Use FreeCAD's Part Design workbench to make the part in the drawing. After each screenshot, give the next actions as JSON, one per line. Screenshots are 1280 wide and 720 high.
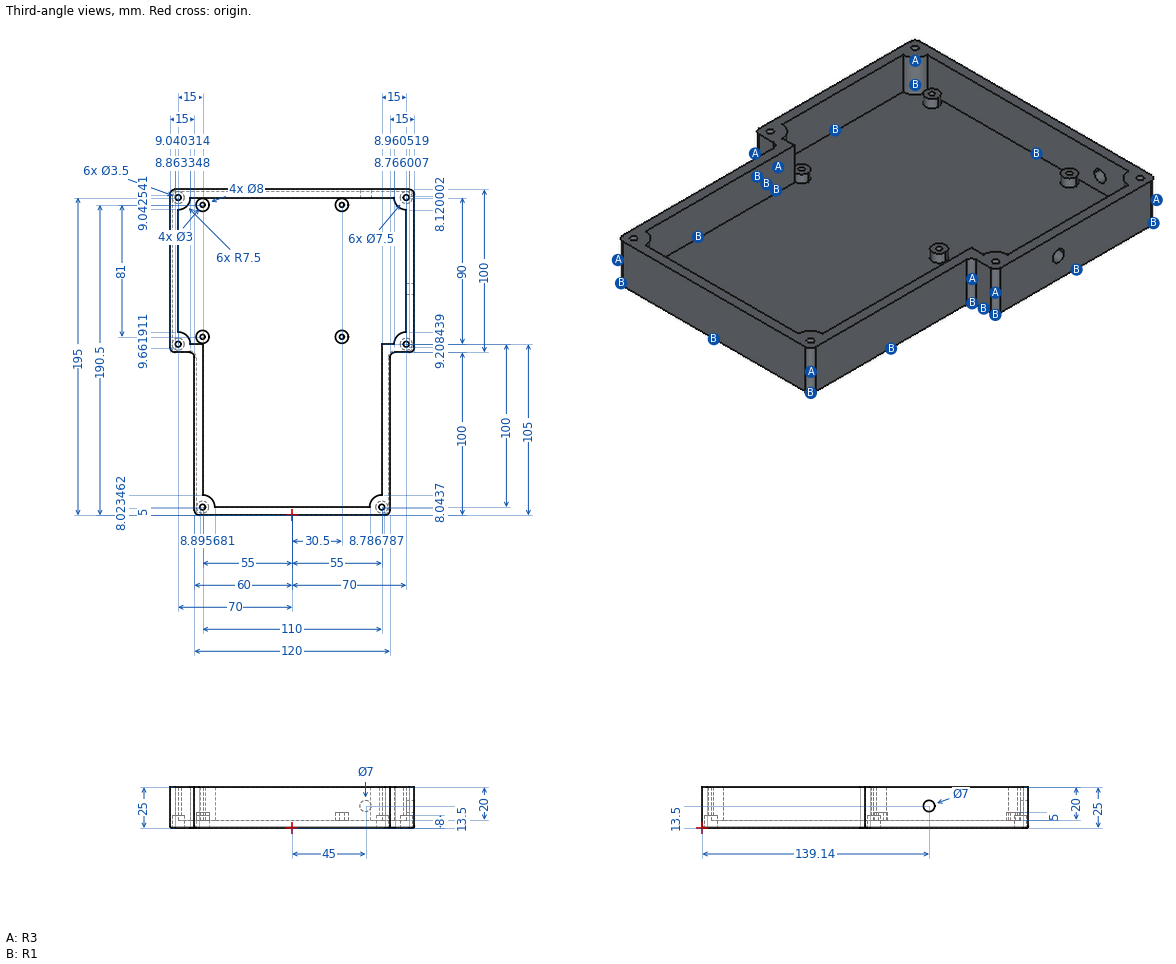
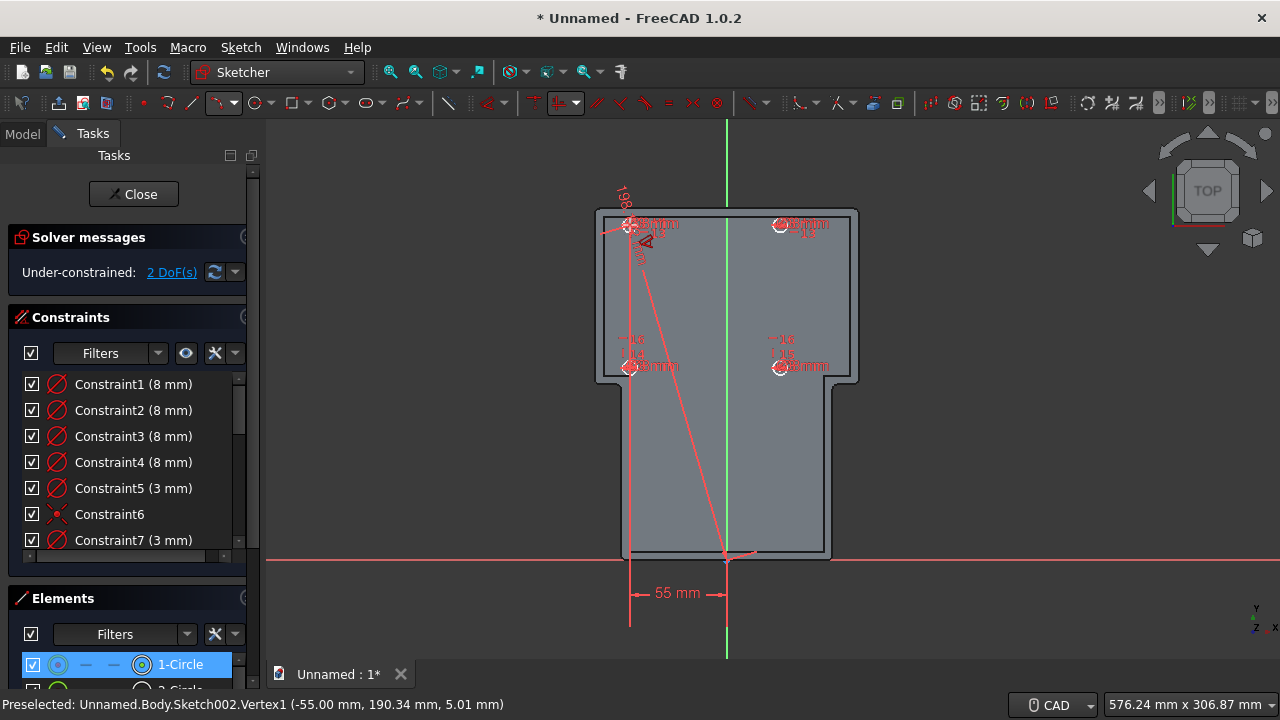
{"action": "left_click", "coordinate": [630, 368]}
{"action": "left_click", "coordinate": [596, 297]}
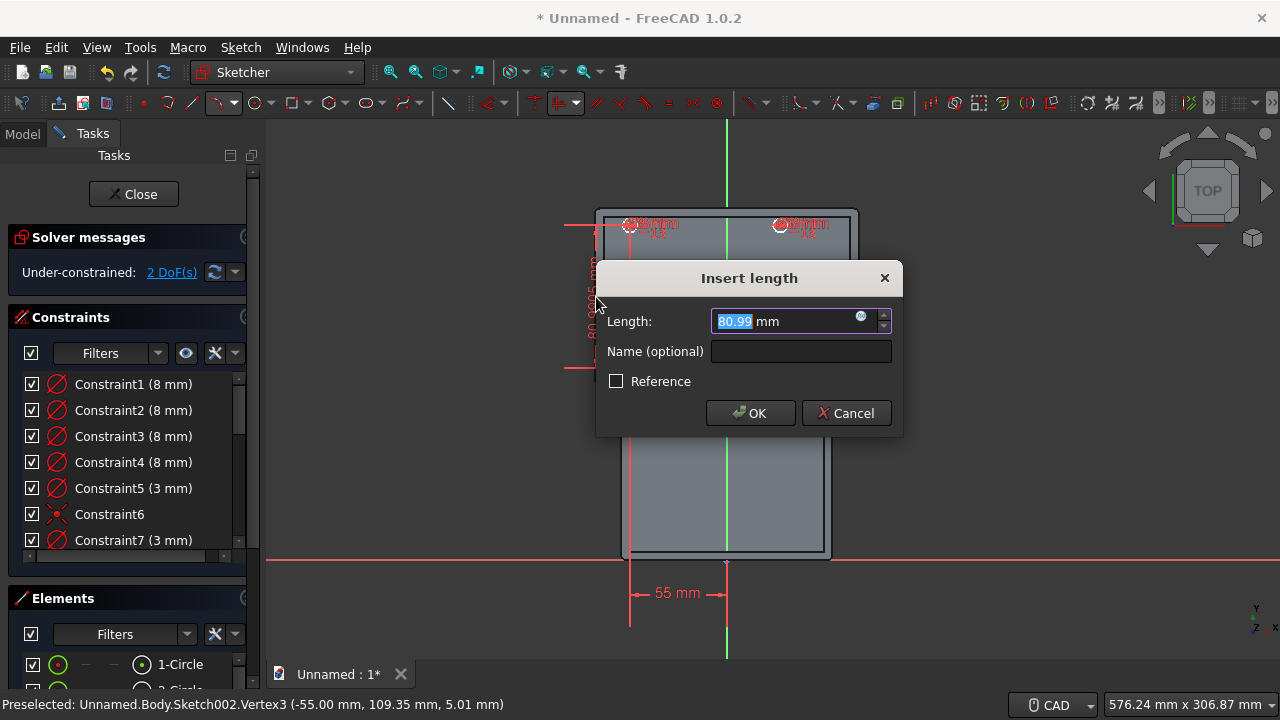
{"action": "type", "text": "81"}
{"action": "key", "text": "Return"}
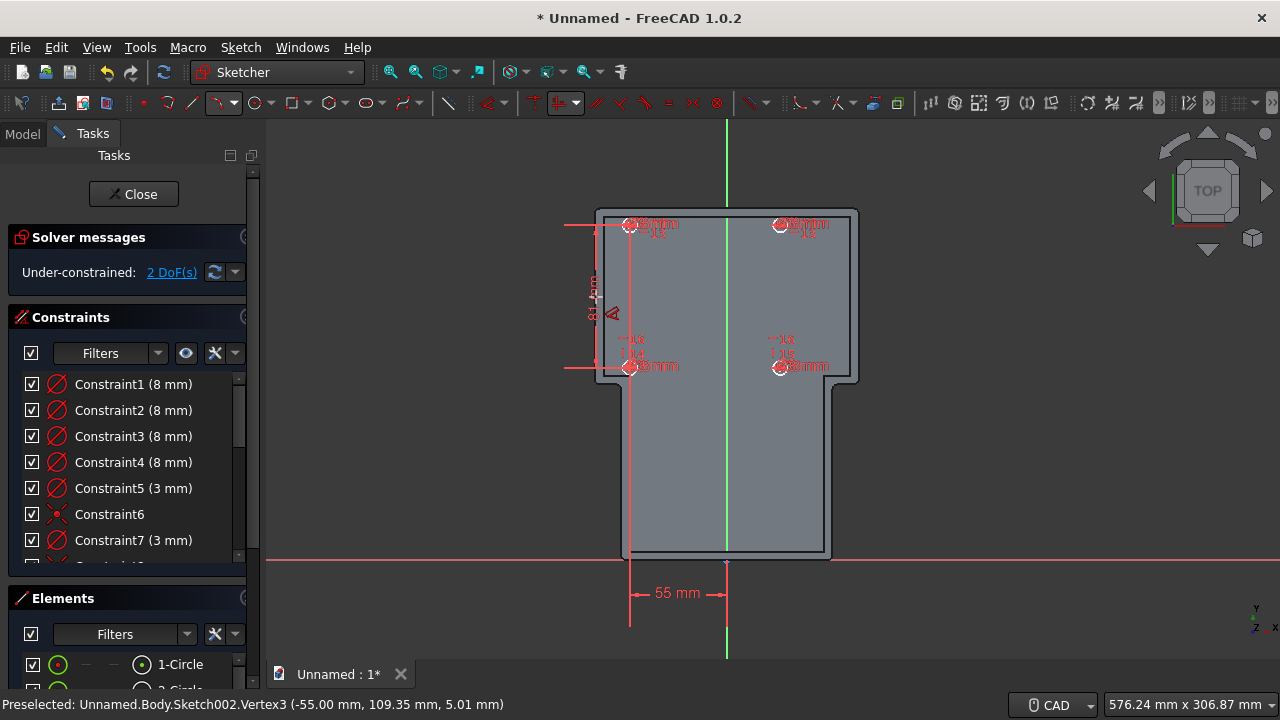
{"action": "left_click", "coordinate": [780, 225]}
{"action": "left_click", "coordinate": [754, 594]}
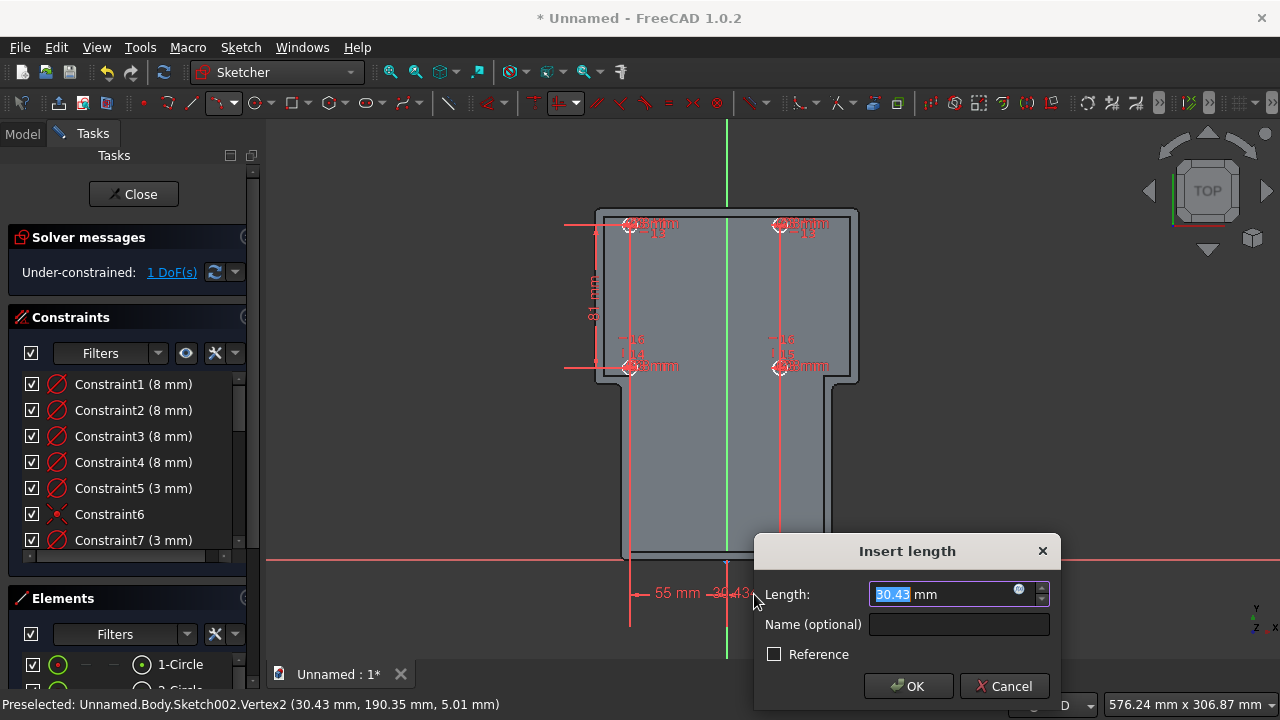
{"action": "type", "text": "30.5"}
{"action": "key", "text": "Return"}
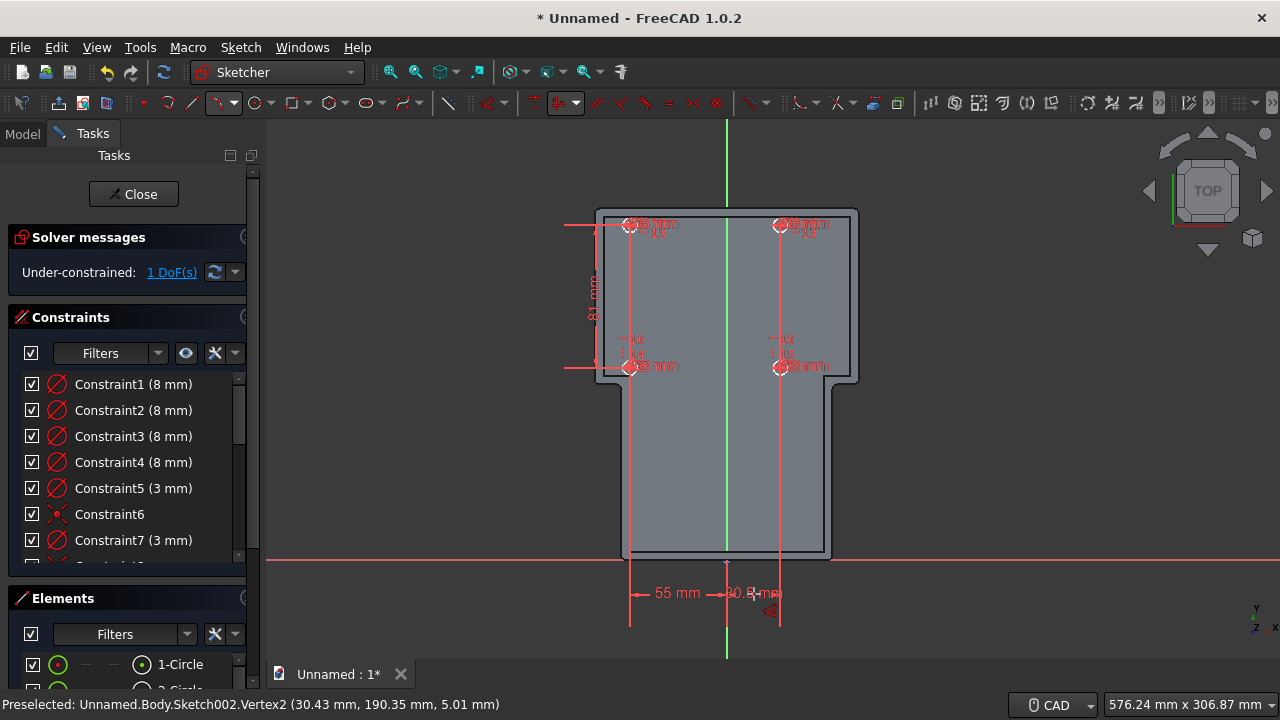
{"action": "left_click", "coordinate": [630, 225]}
{"action": "left_click", "coordinate": [596, 393]}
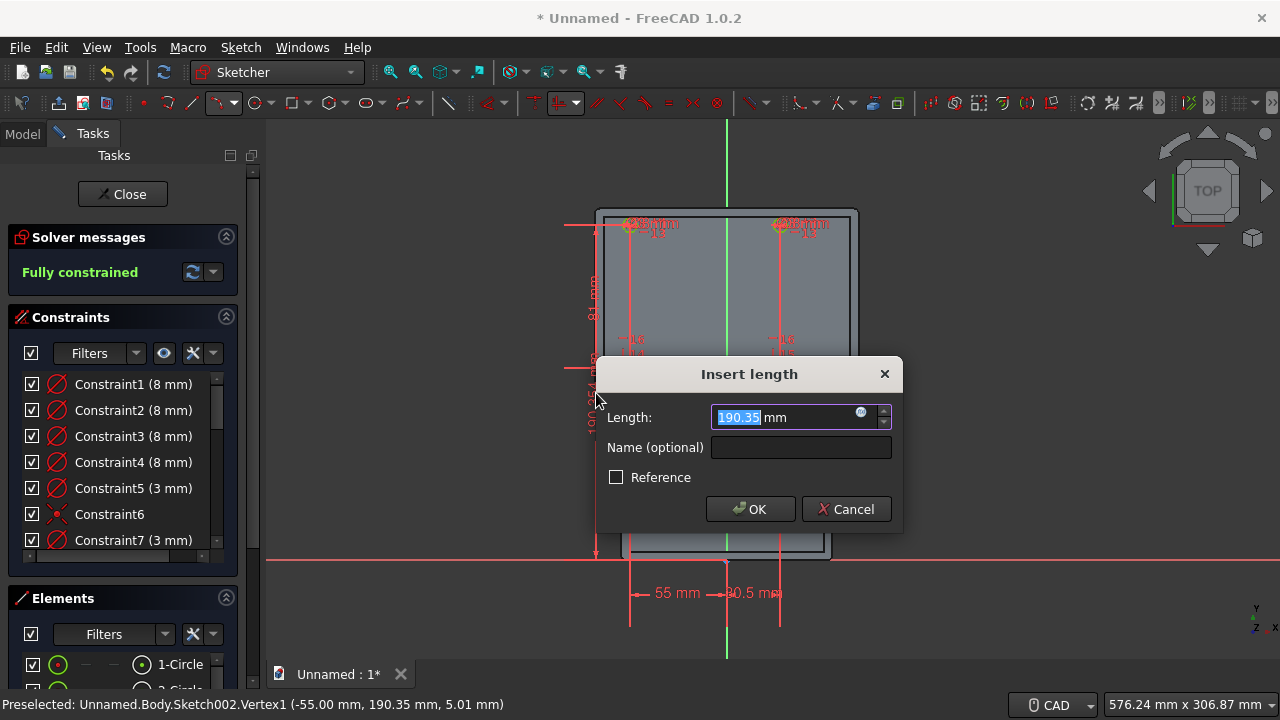
{"action": "type", "text": "190.5"}
{"action": "key", "text": "Return"}
{"action": "key", "text": "Escape"}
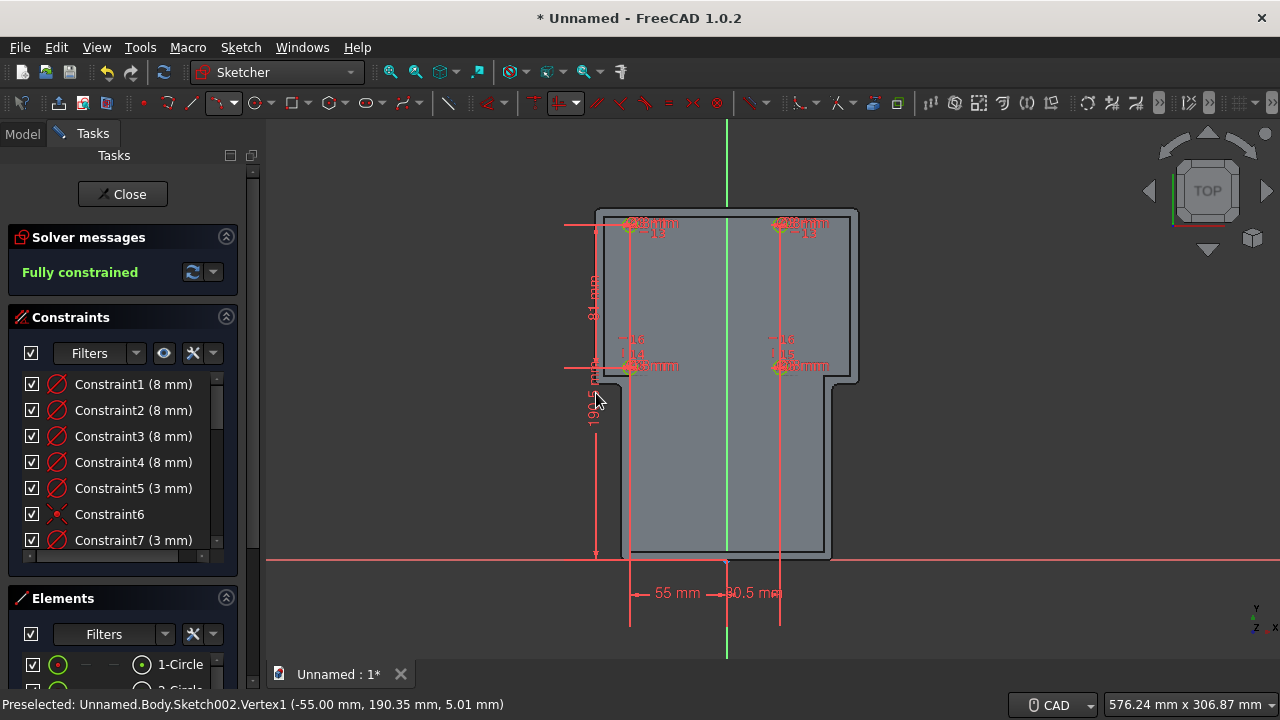
{"action": "left_click", "coordinate": [123, 194]}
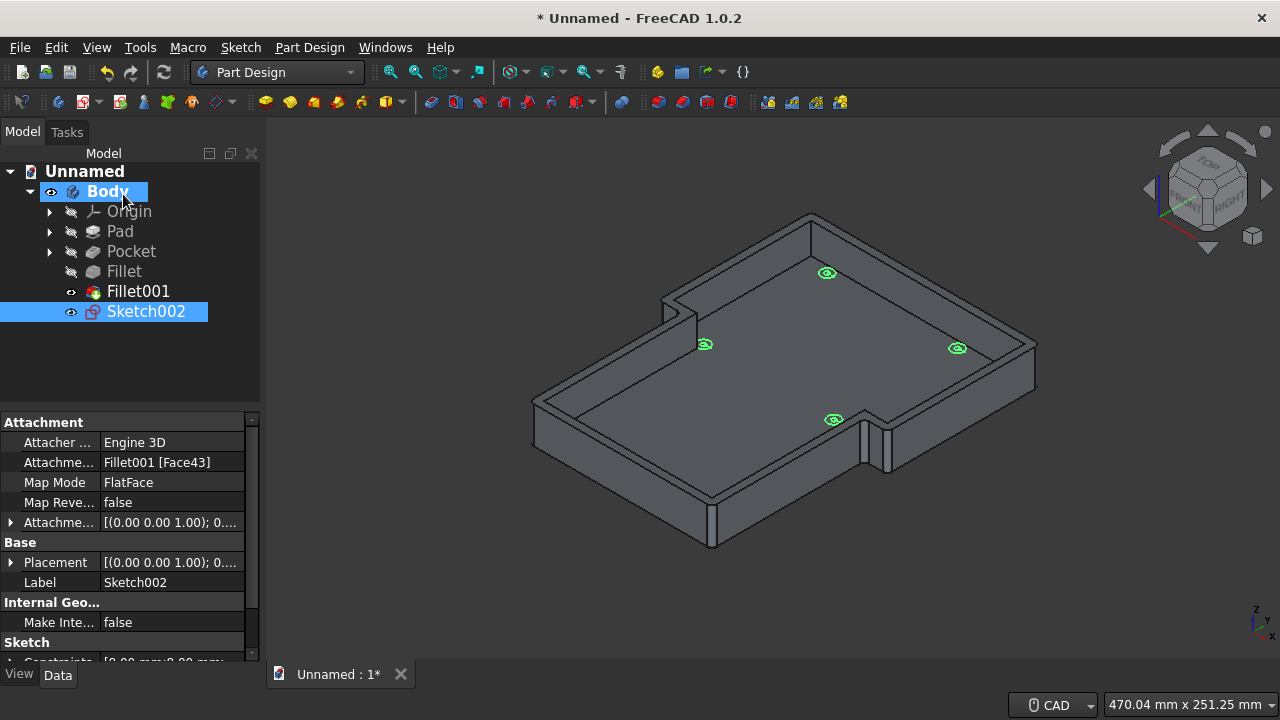
{"action": "left_click", "coordinate": [266, 102]}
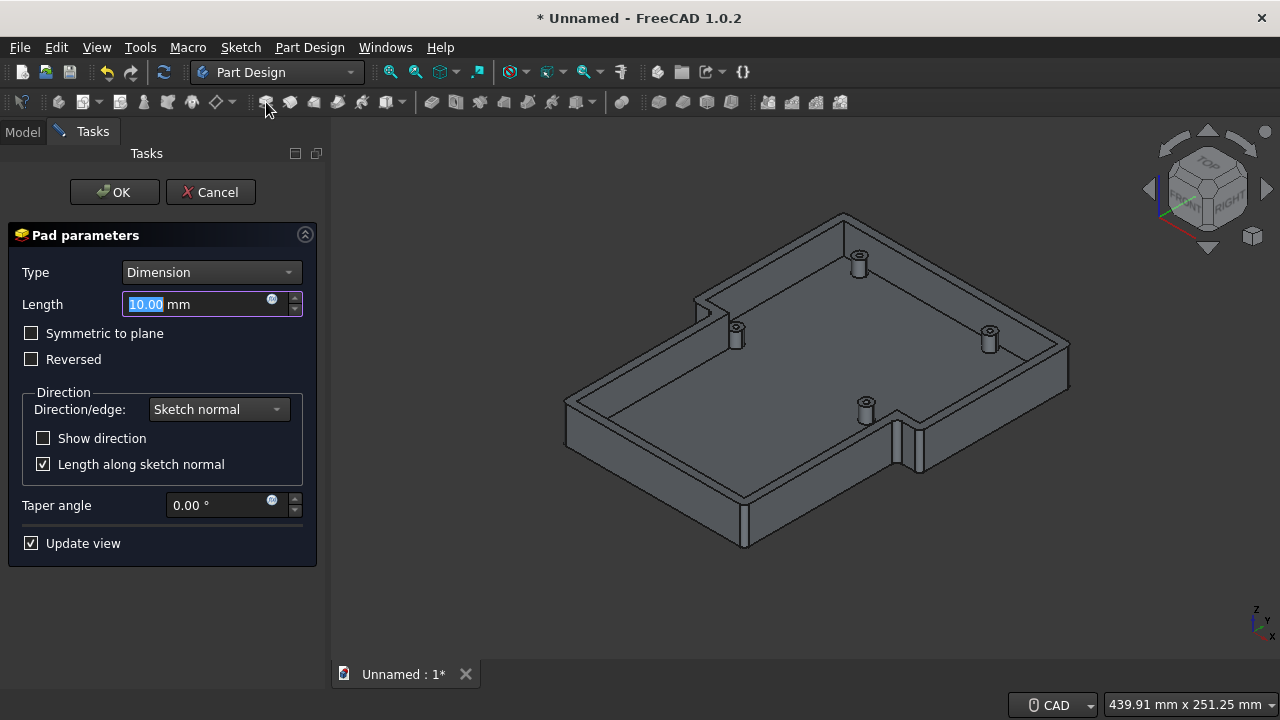
{"action": "type", "text": "5"}
{"action": "key", "text": "Tab"}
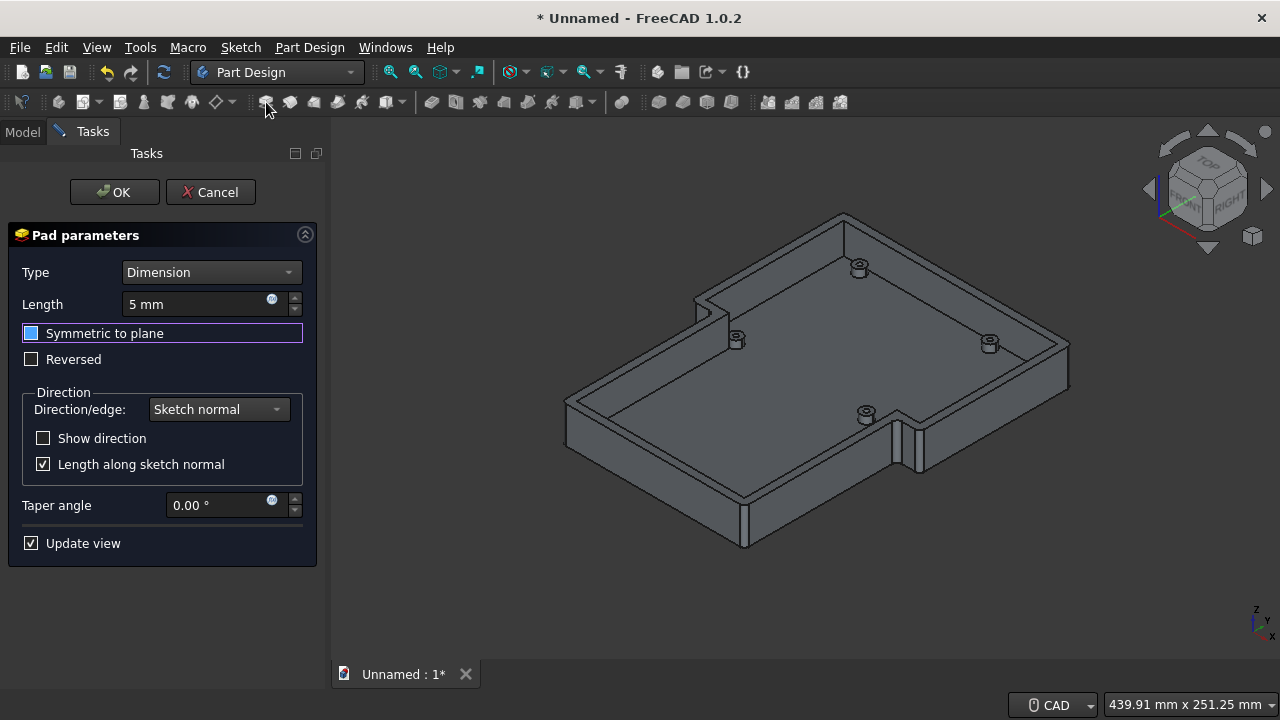
{"action": "left_click", "coordinate": [115, 192]}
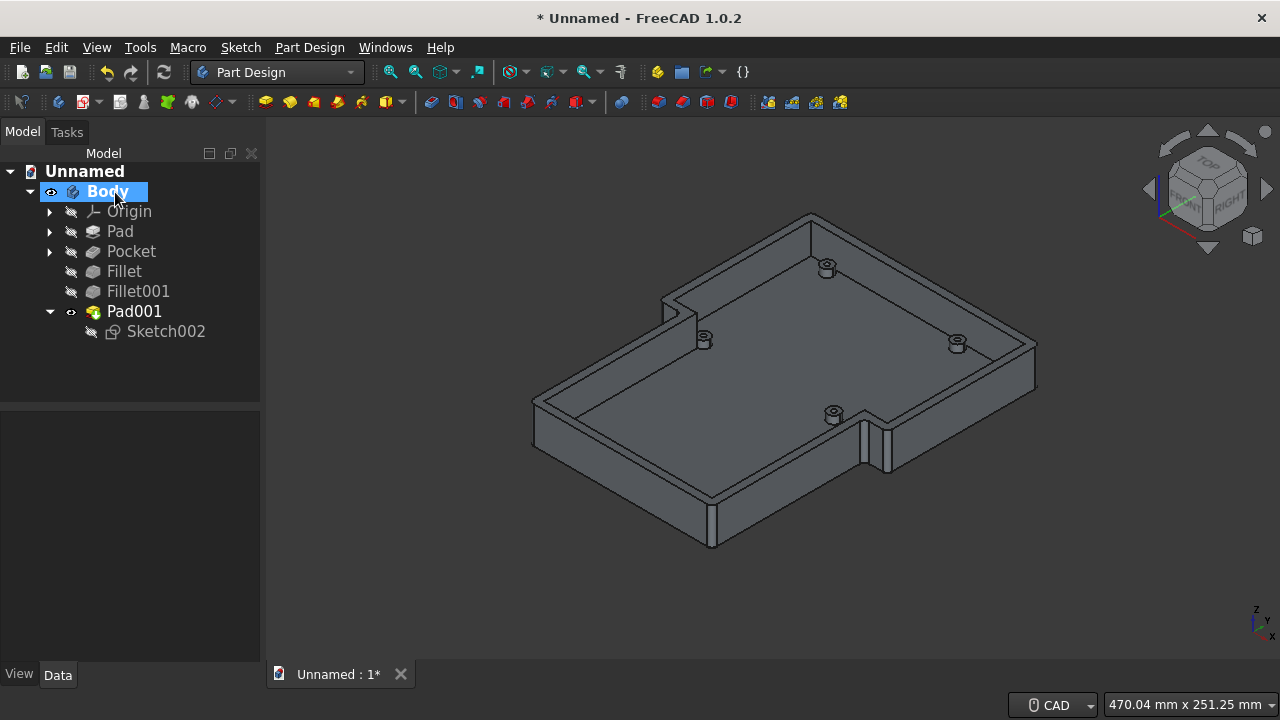
{"action": "scroll", "coordinate": [685, 312], "scroll_direction": "up", "scroll_amount": 4}